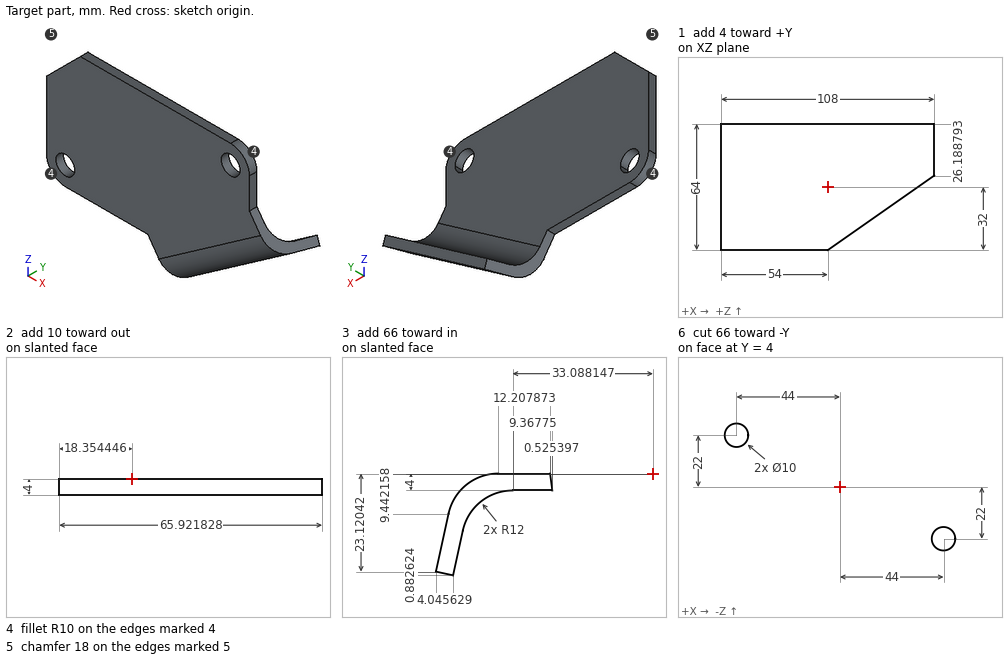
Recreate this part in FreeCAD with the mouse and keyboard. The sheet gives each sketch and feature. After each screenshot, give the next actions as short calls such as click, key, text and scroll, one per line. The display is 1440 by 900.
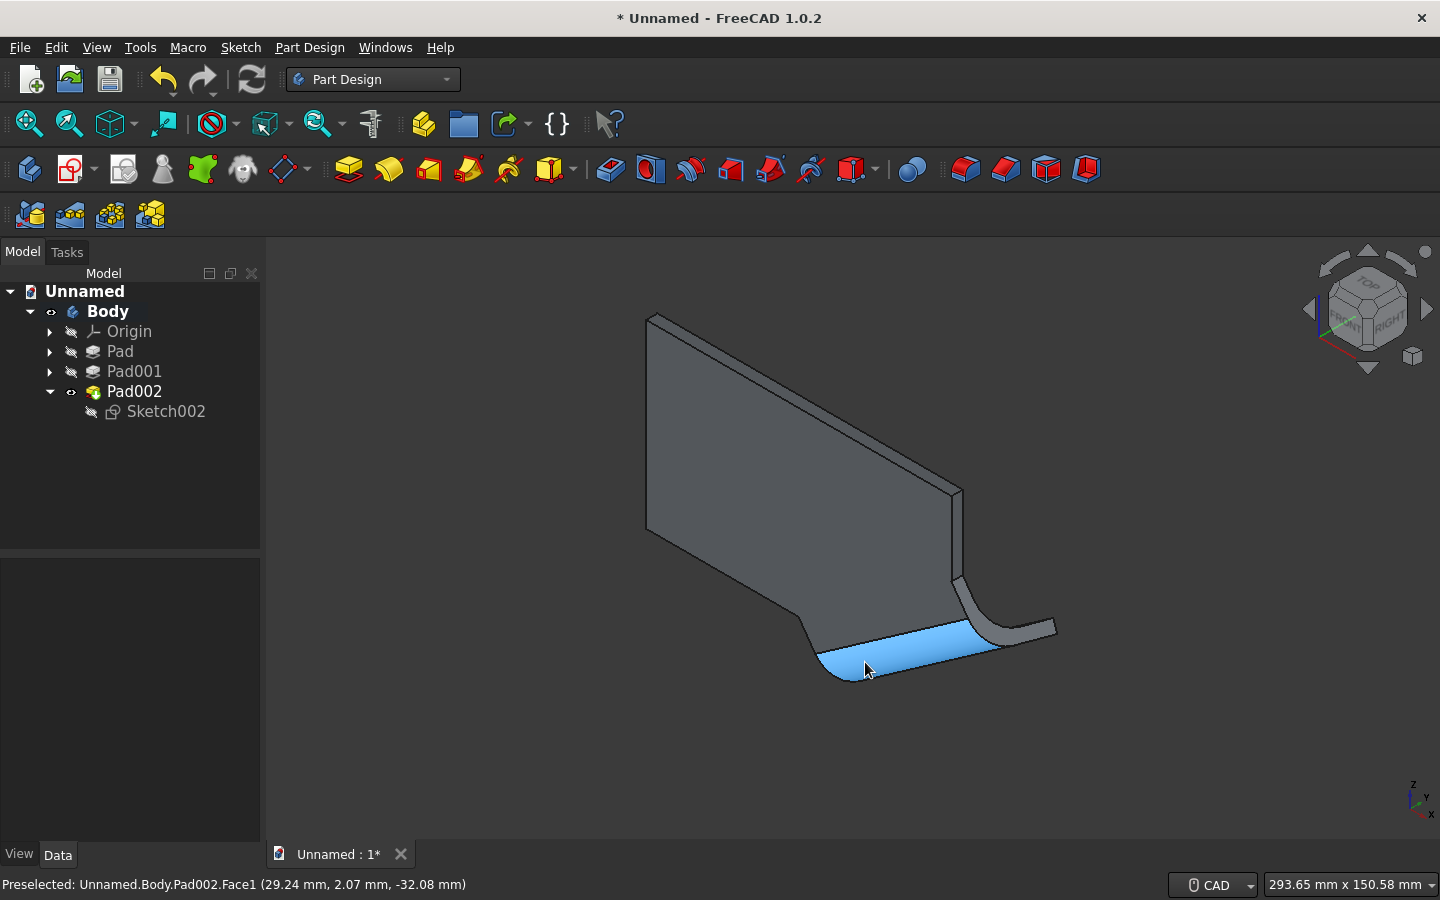
click(958, 491)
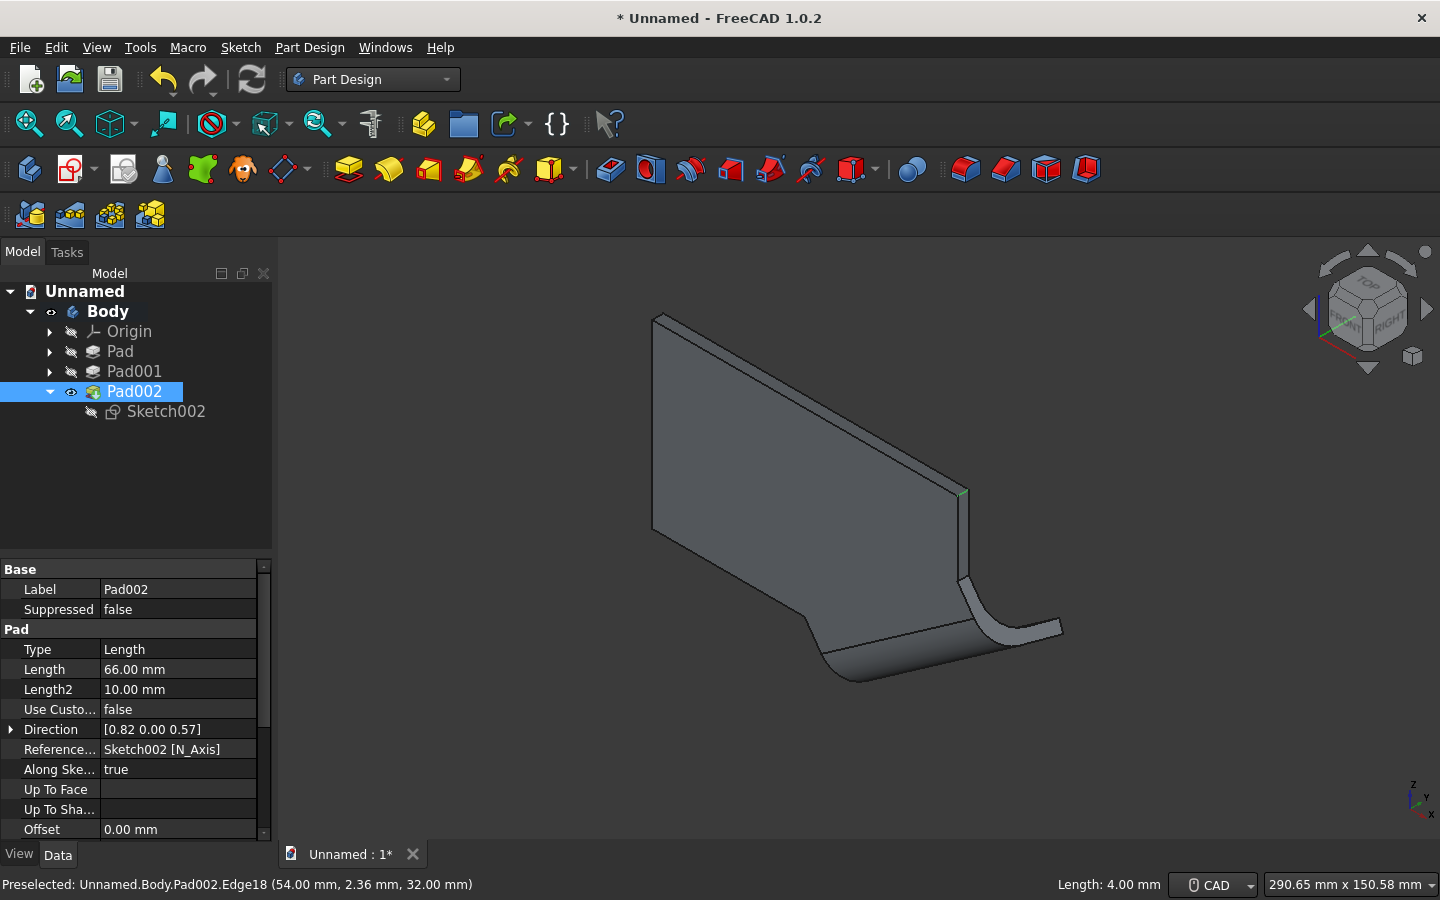
scroll(658, 525, up, 5)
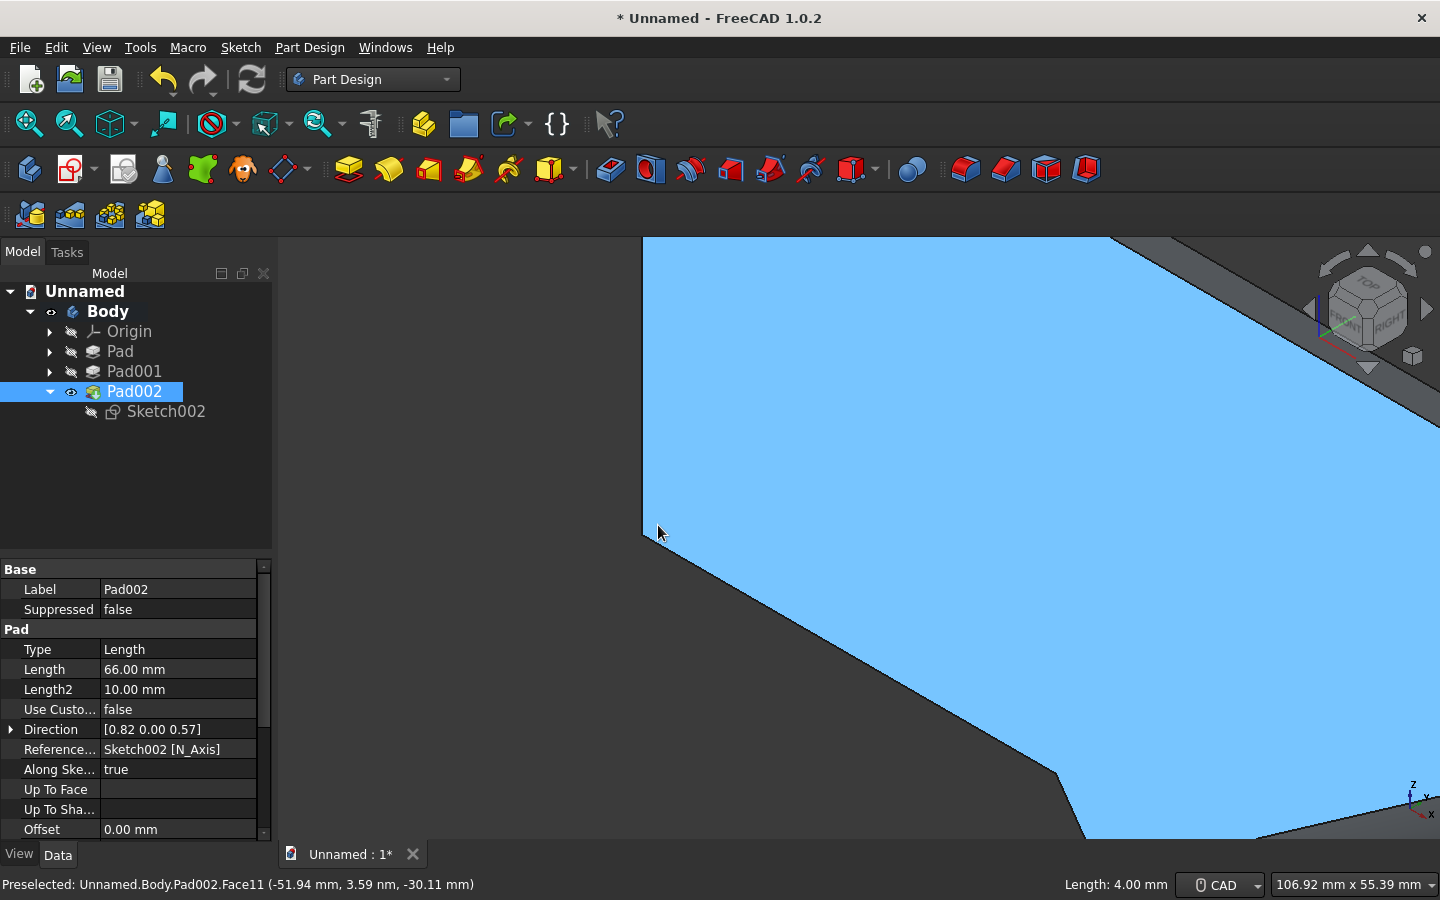
key(v)
key(f)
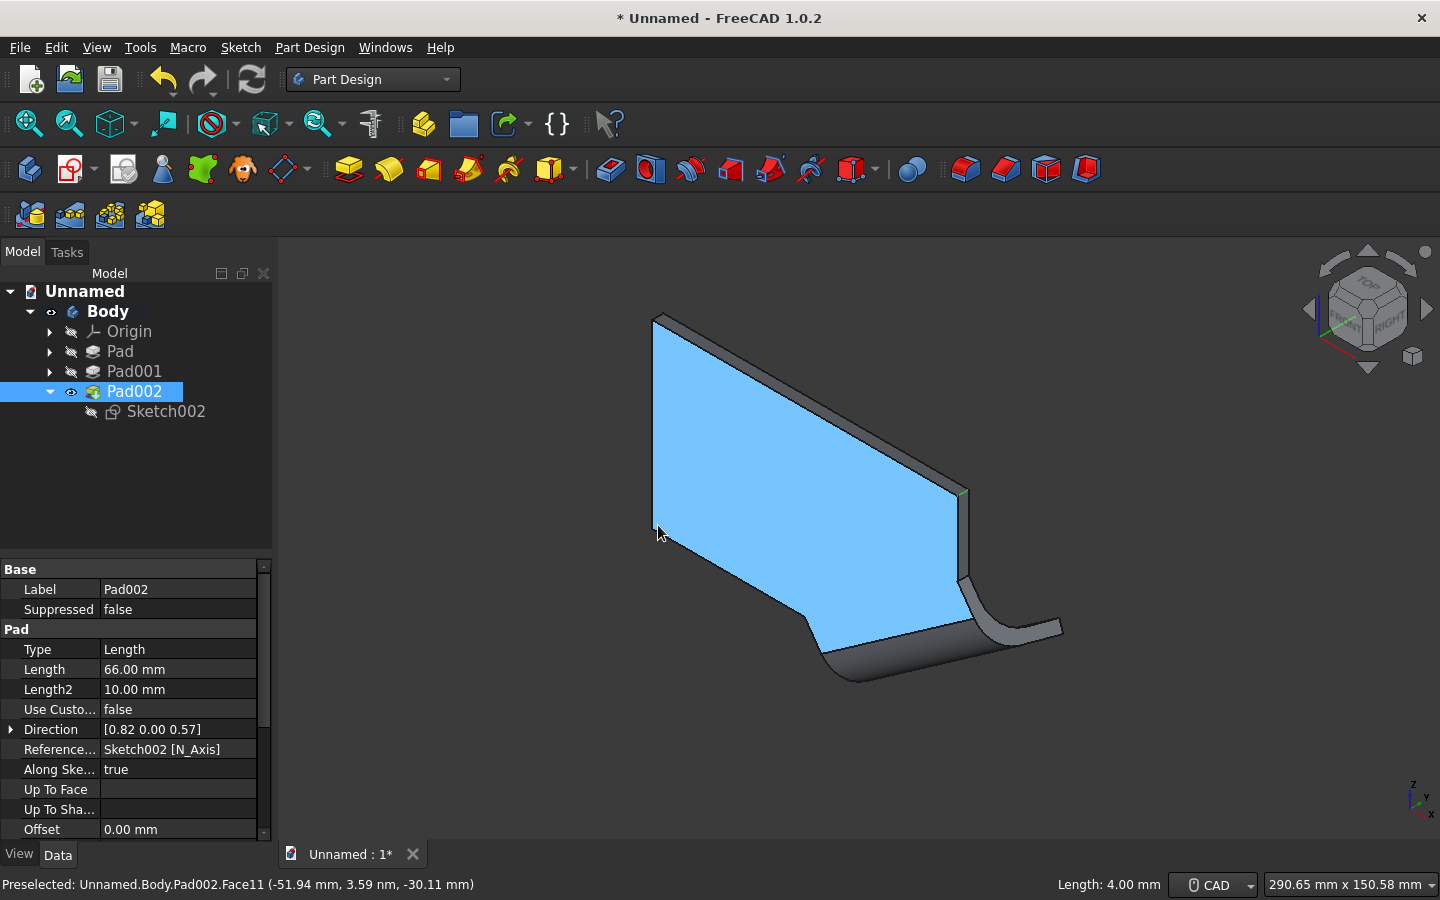
key(2)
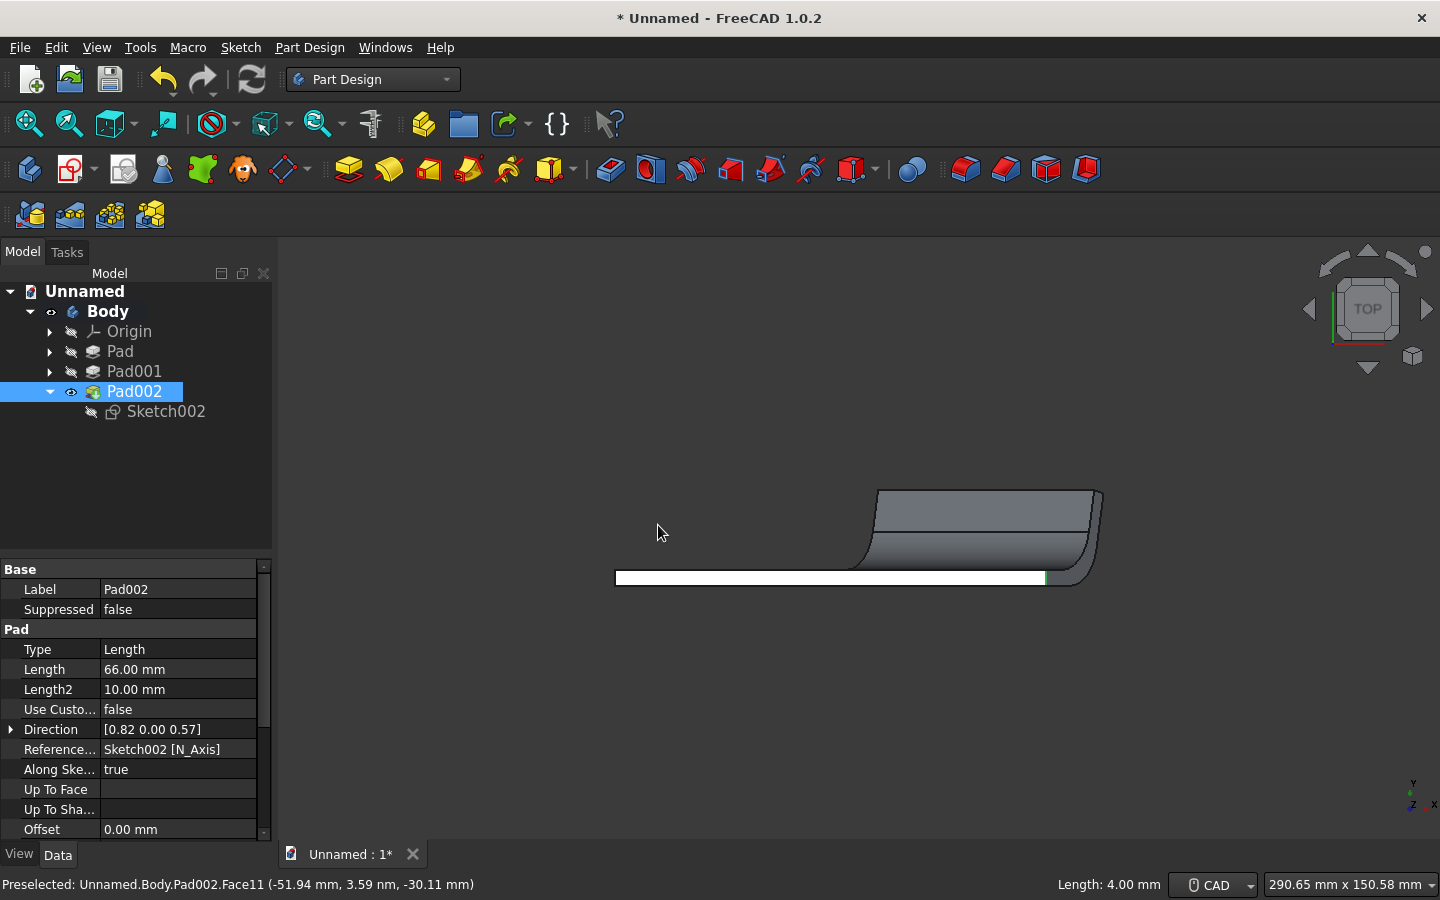
key(v)
key(f)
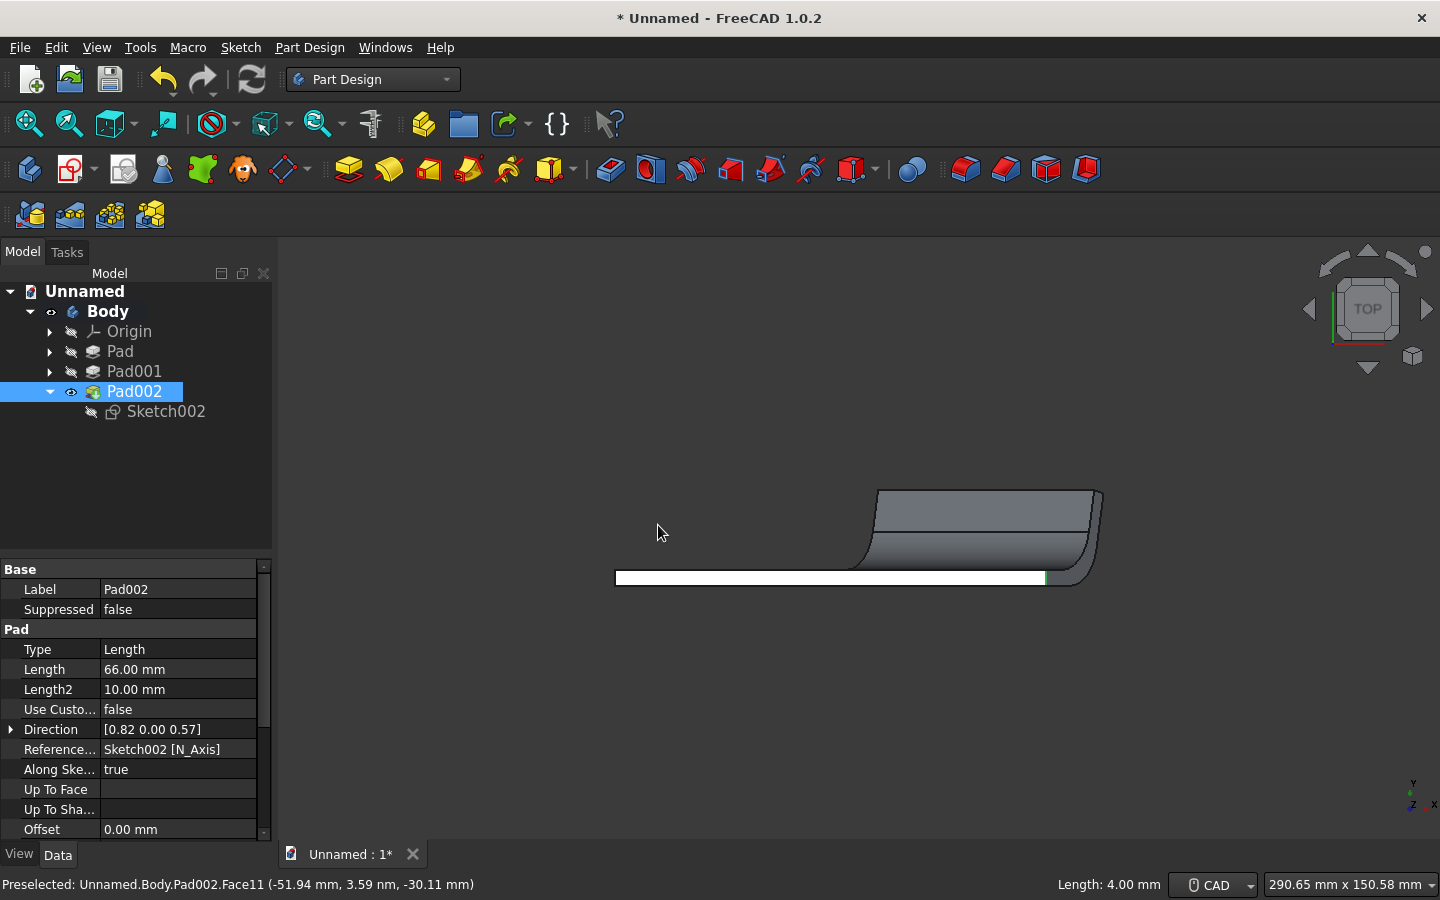
scroll(615, 577, up, 5)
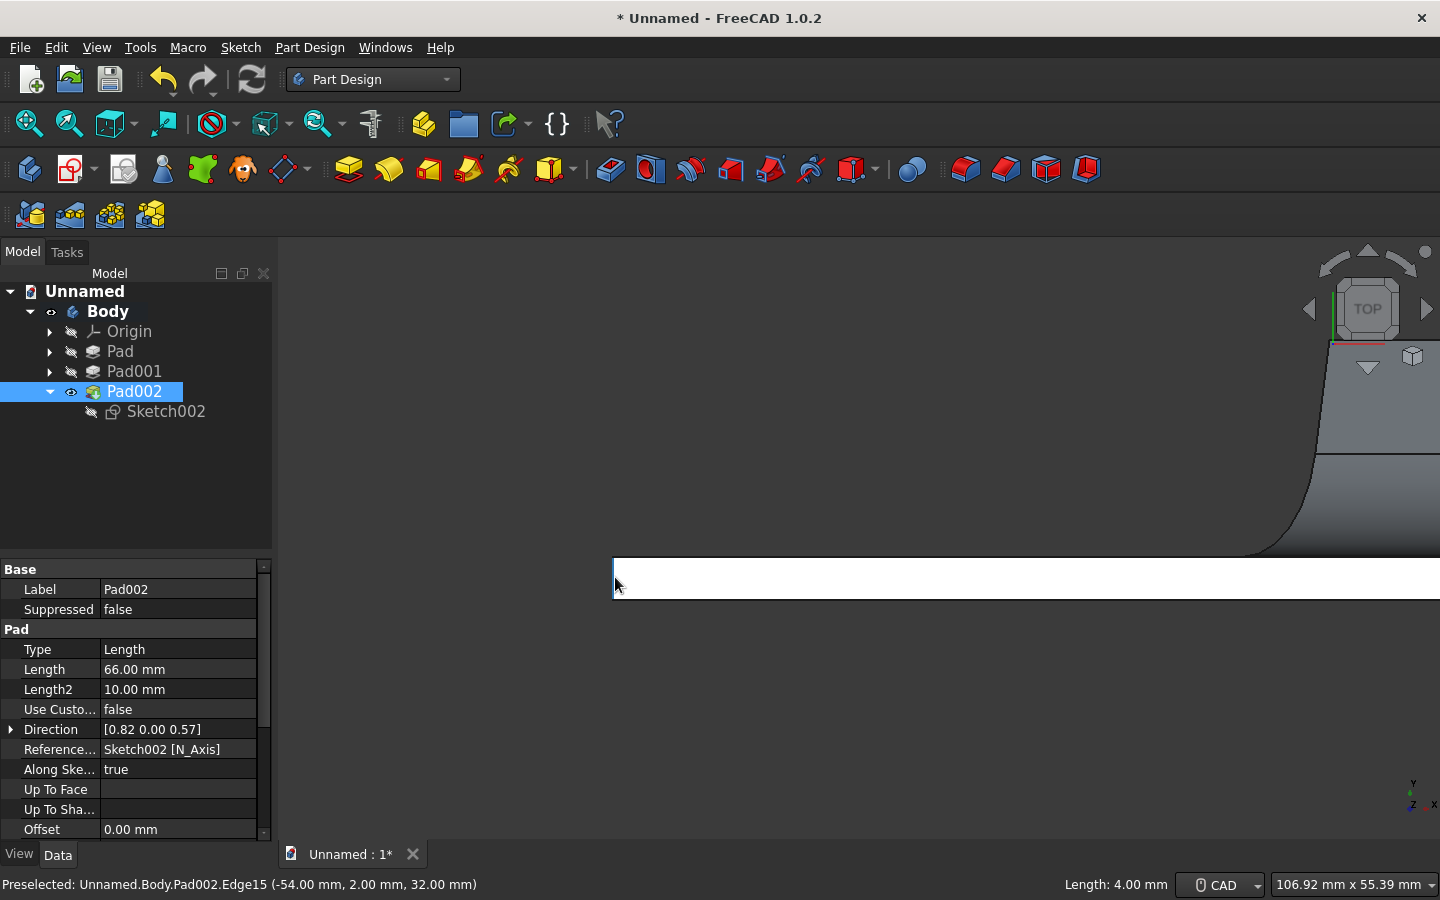
key(v)
key(f)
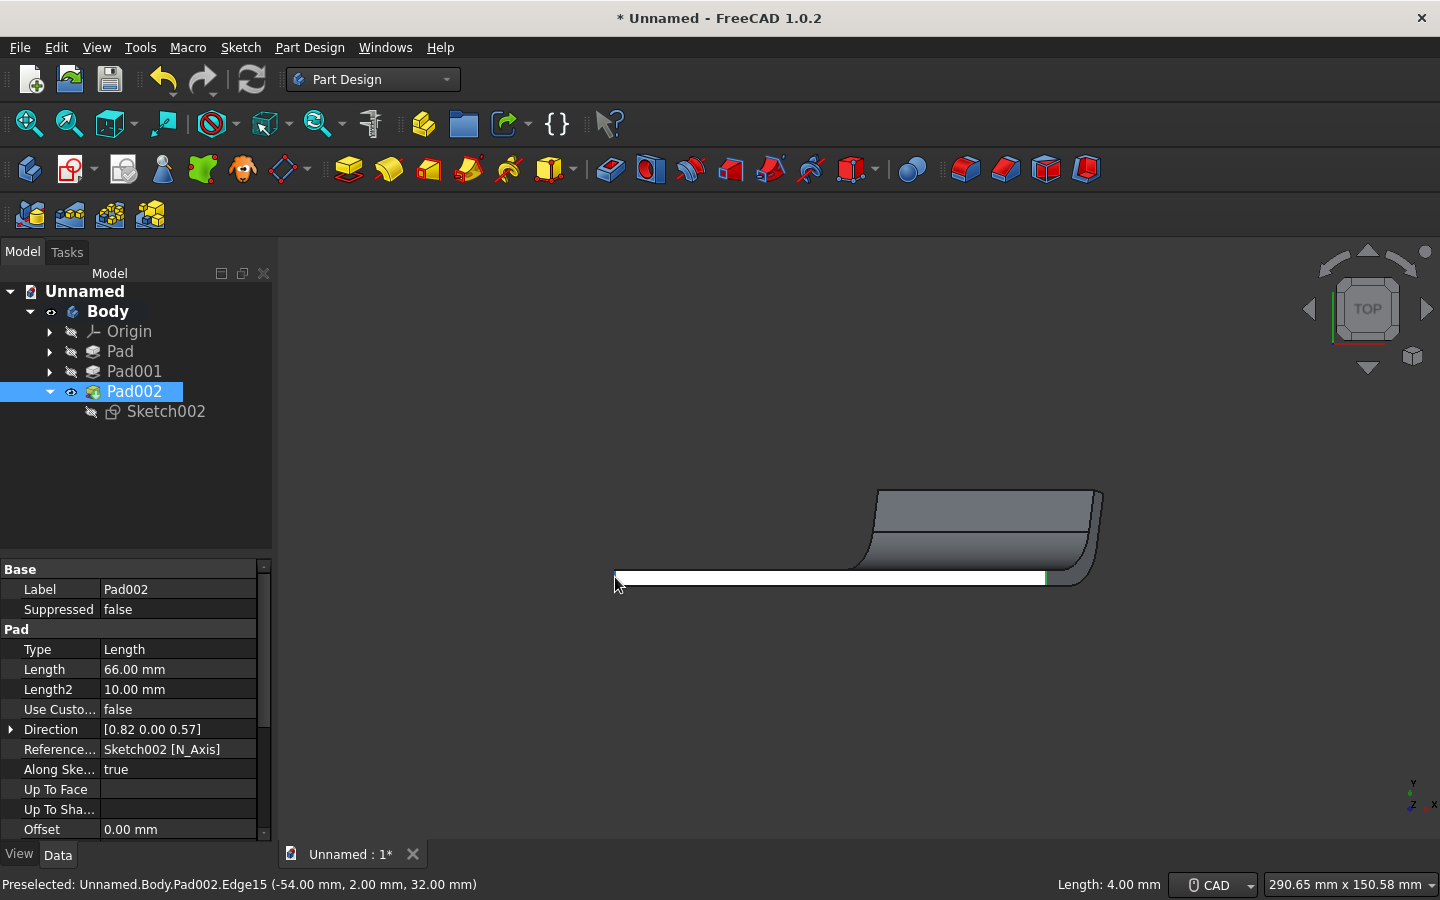
key(1)